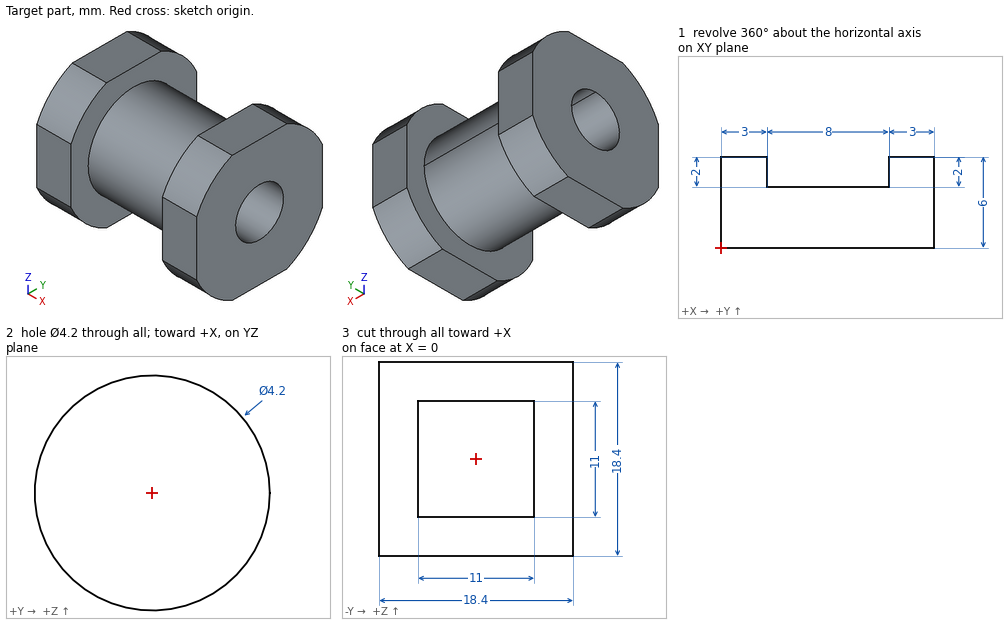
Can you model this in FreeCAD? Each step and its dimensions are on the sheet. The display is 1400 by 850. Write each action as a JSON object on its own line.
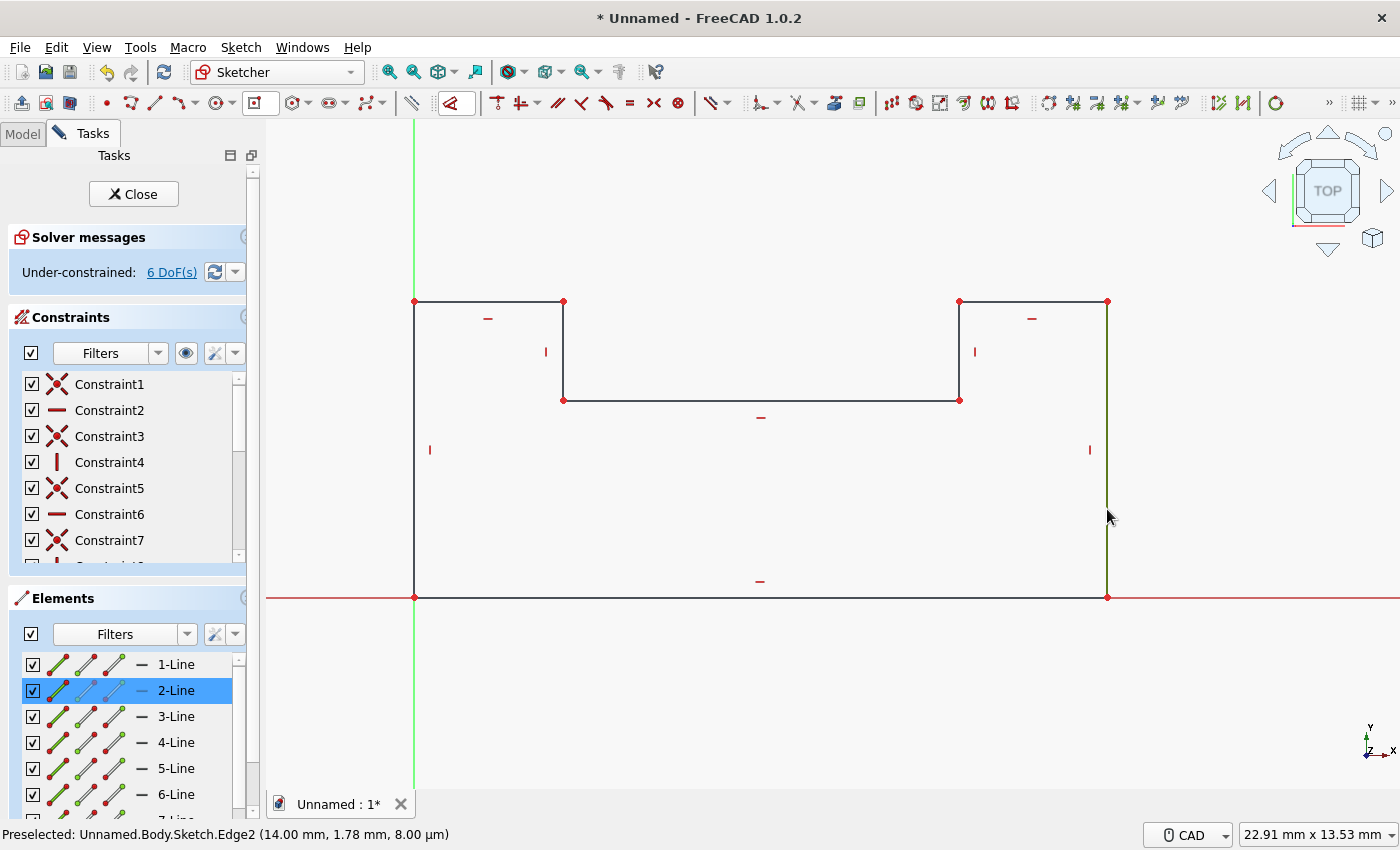
{"action": "left_click", "coordinate": [470, 104]}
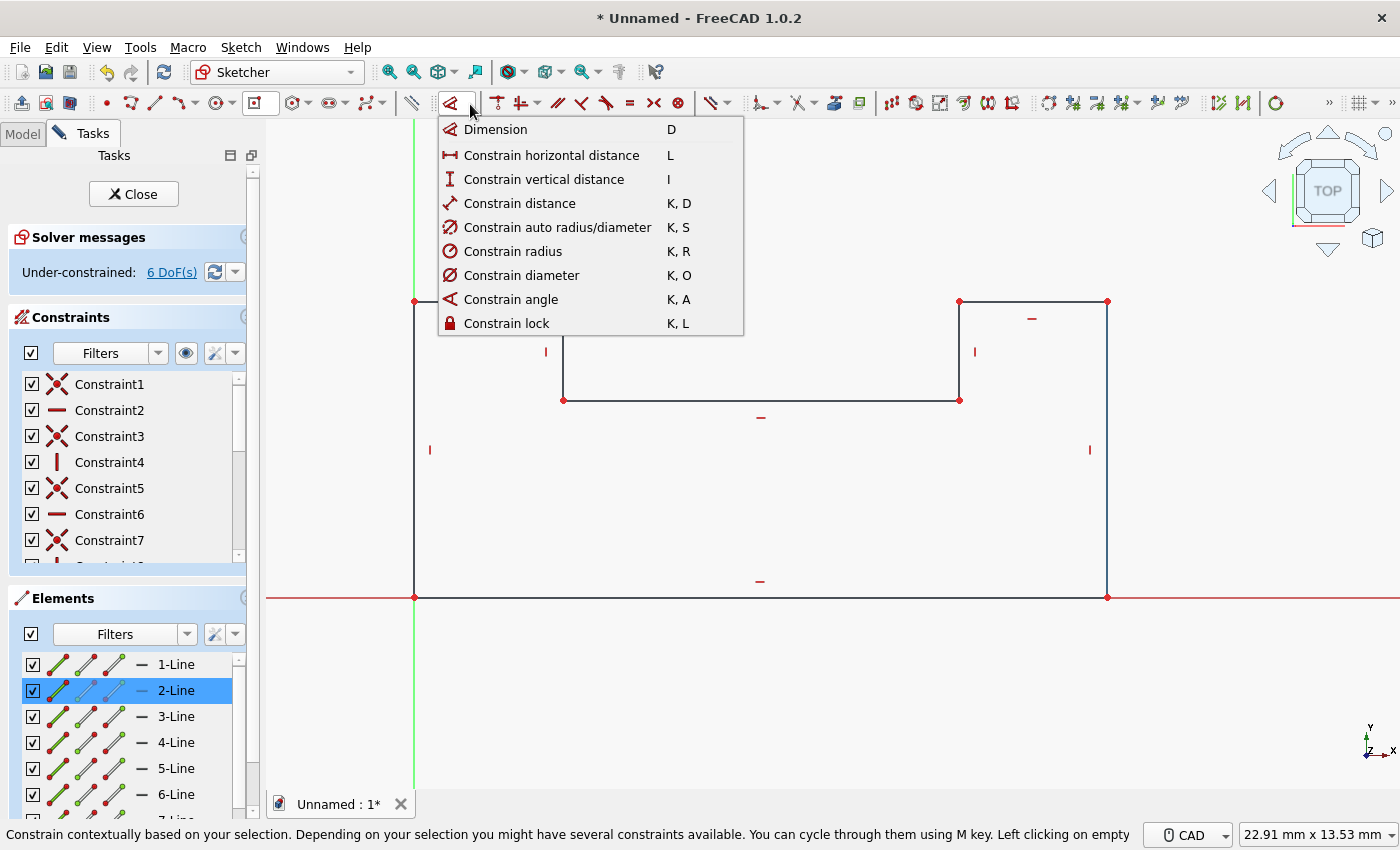
{"action": "left_click", "coordinate": [591, 179]}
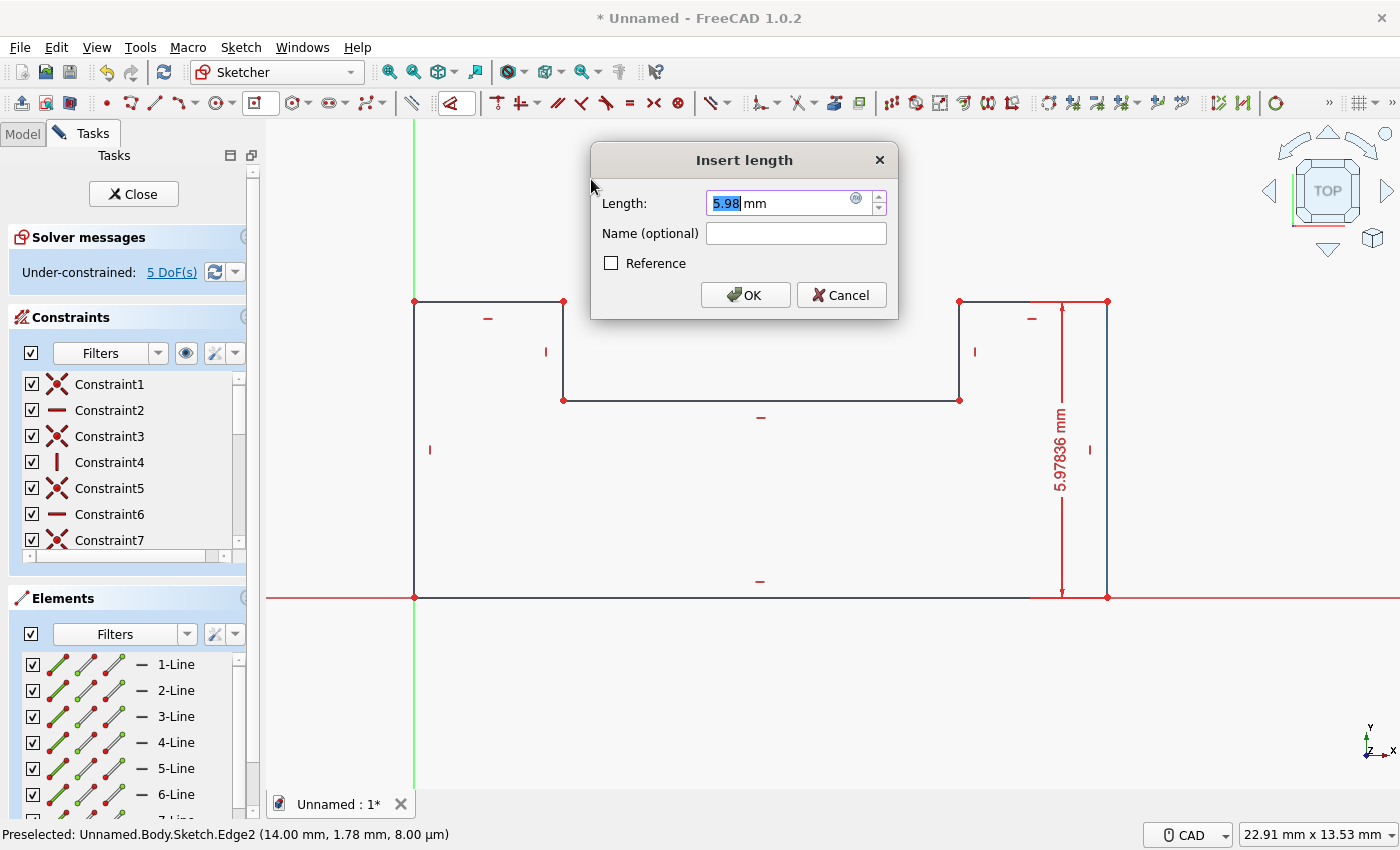
{"action": "type", "text": "6"}
{"action": "key", "text": "Return"}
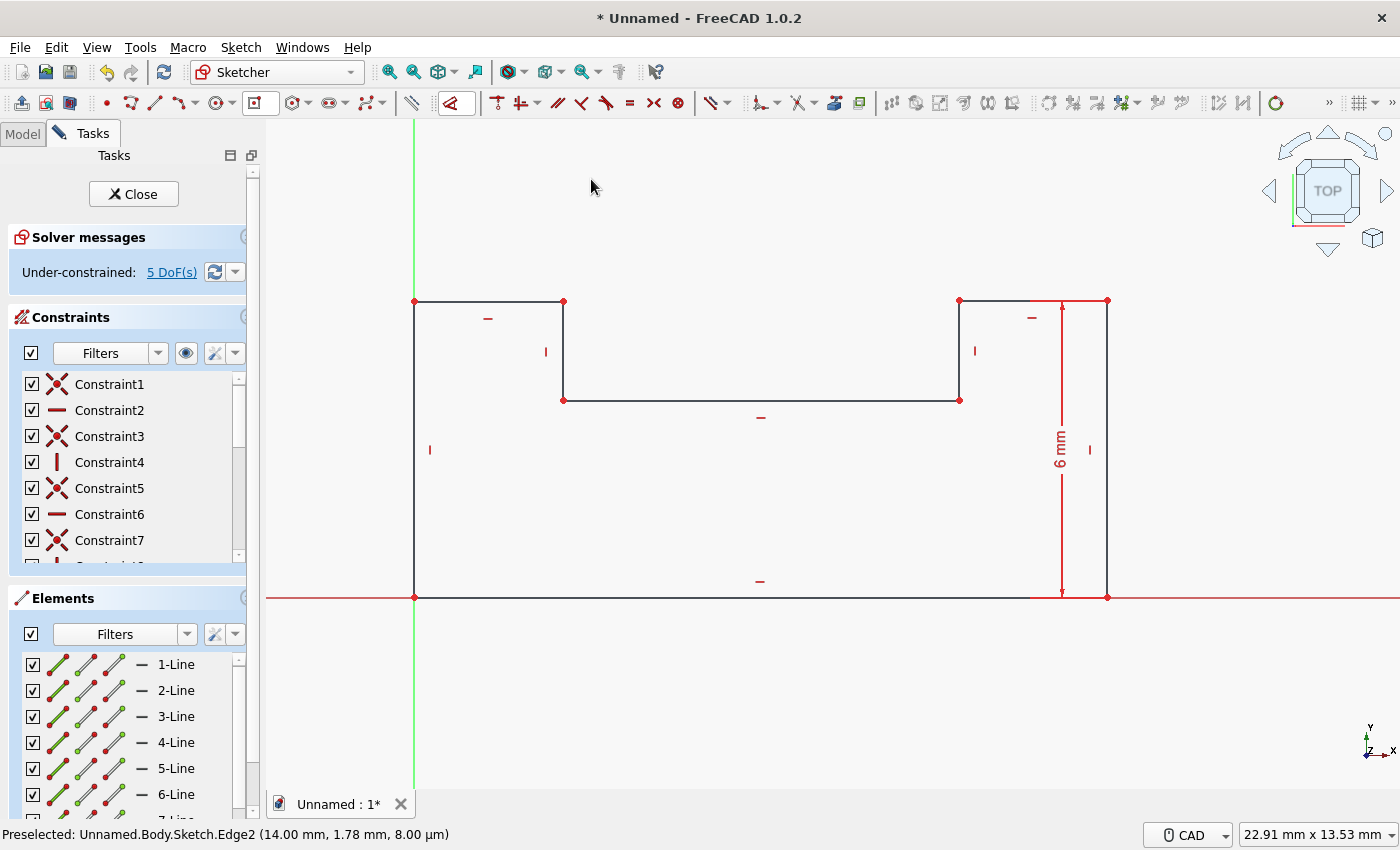
{"action": "left_click", "coordinate": [1063, 301]}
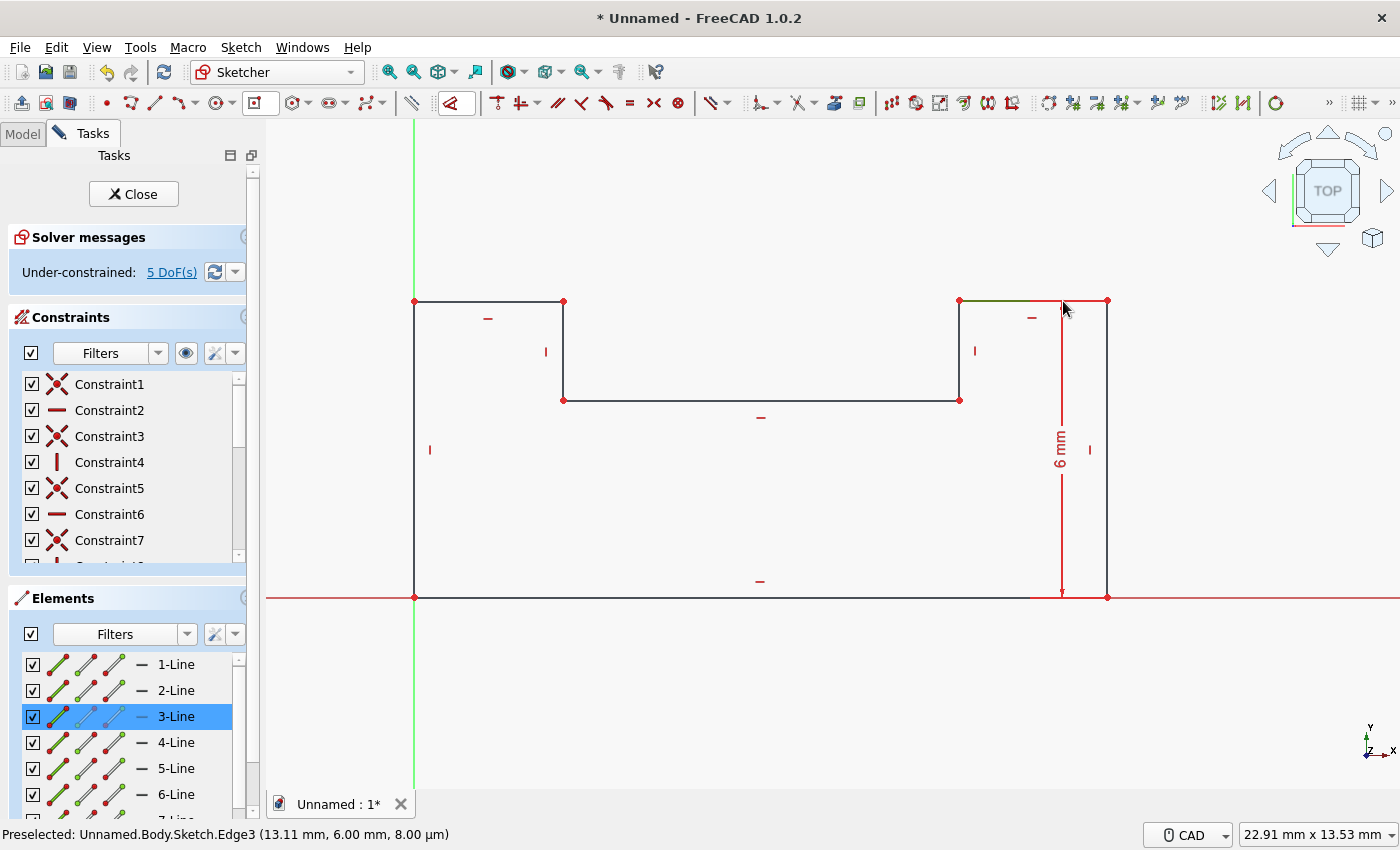
{"action": "left_click", "coordinate": [470, 104]}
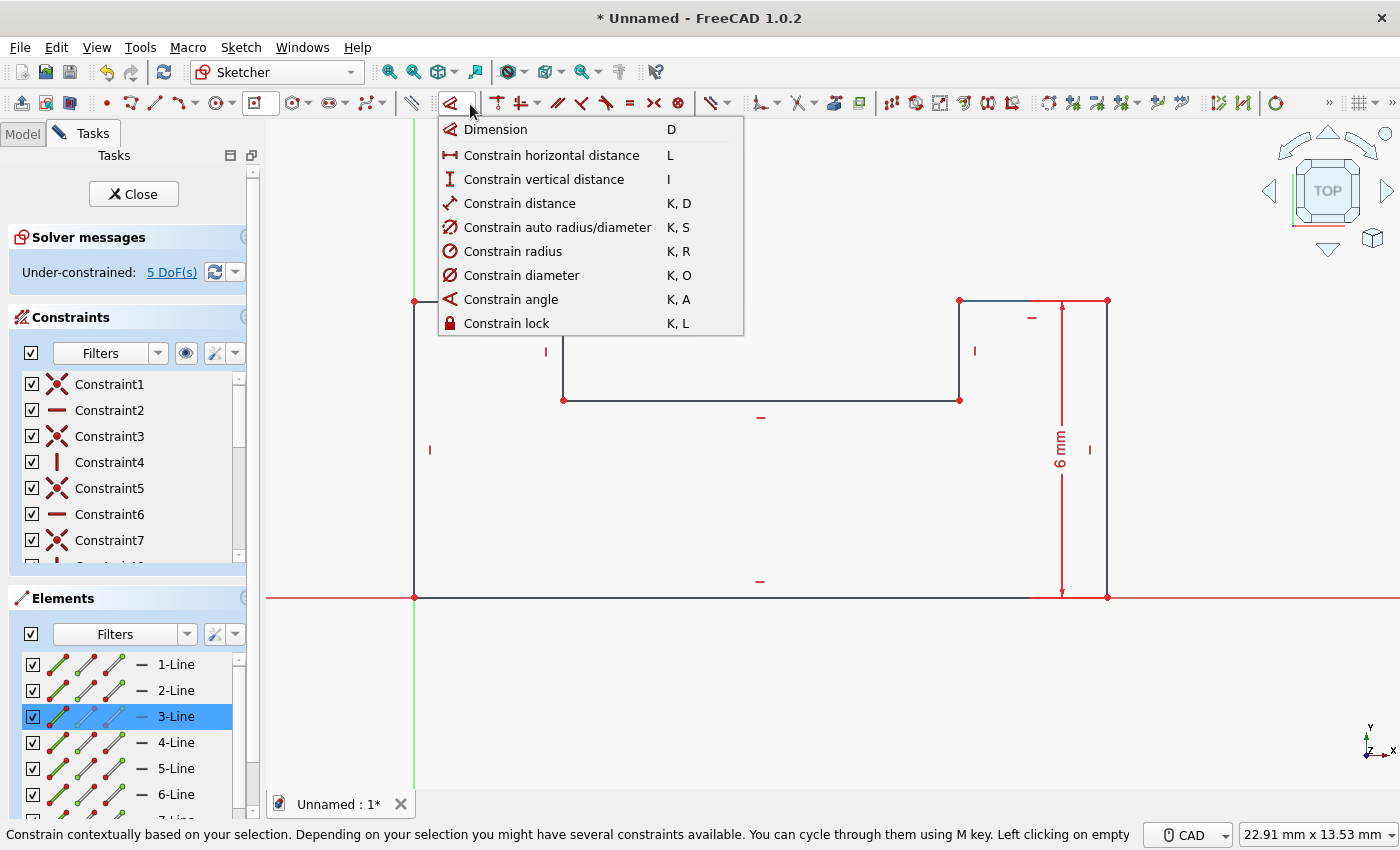
{"action": "left_click", "coordinate": [591, 155]}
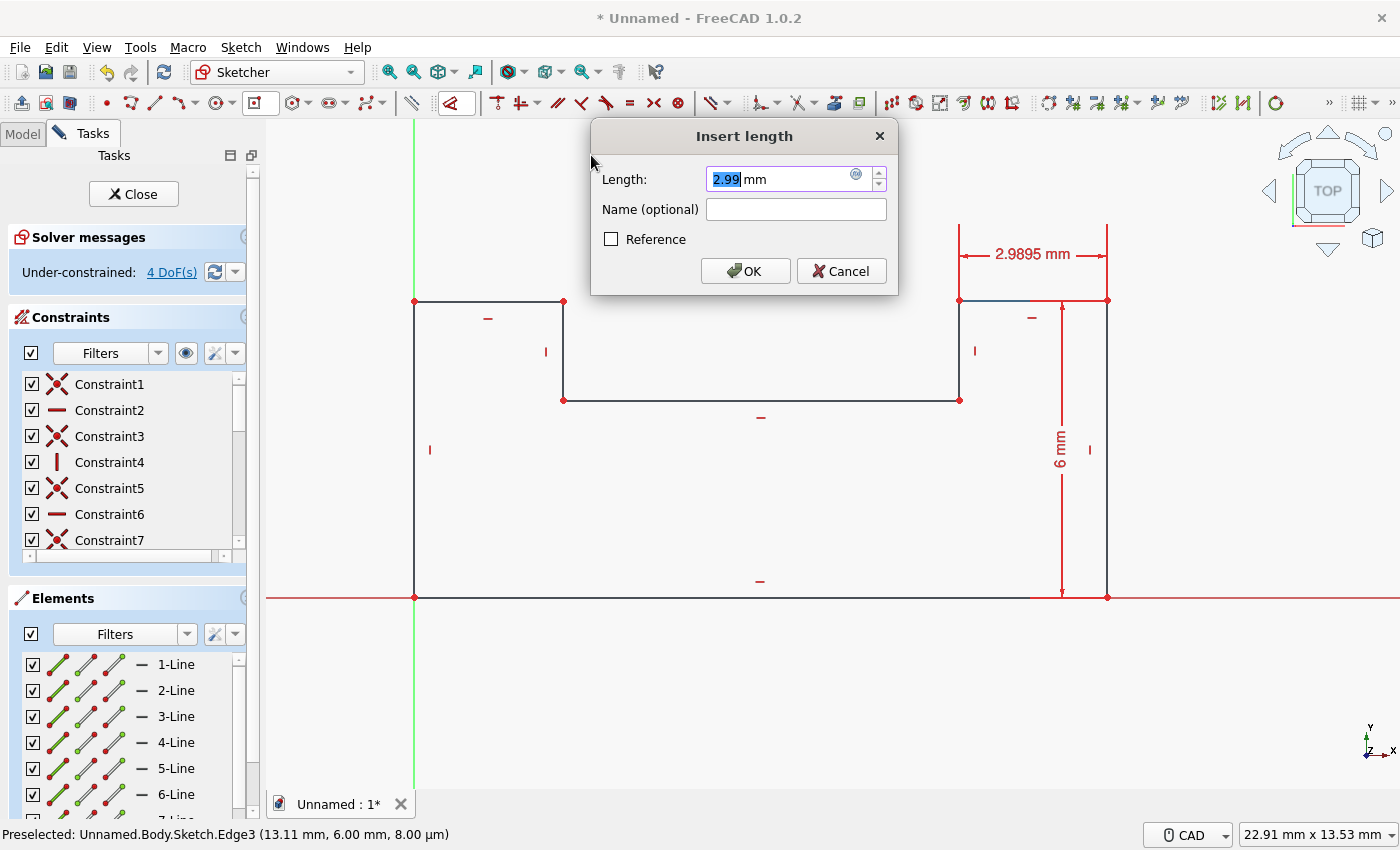
{"action": "type", "text": "3"}
{"action": "key", "text": "Return"}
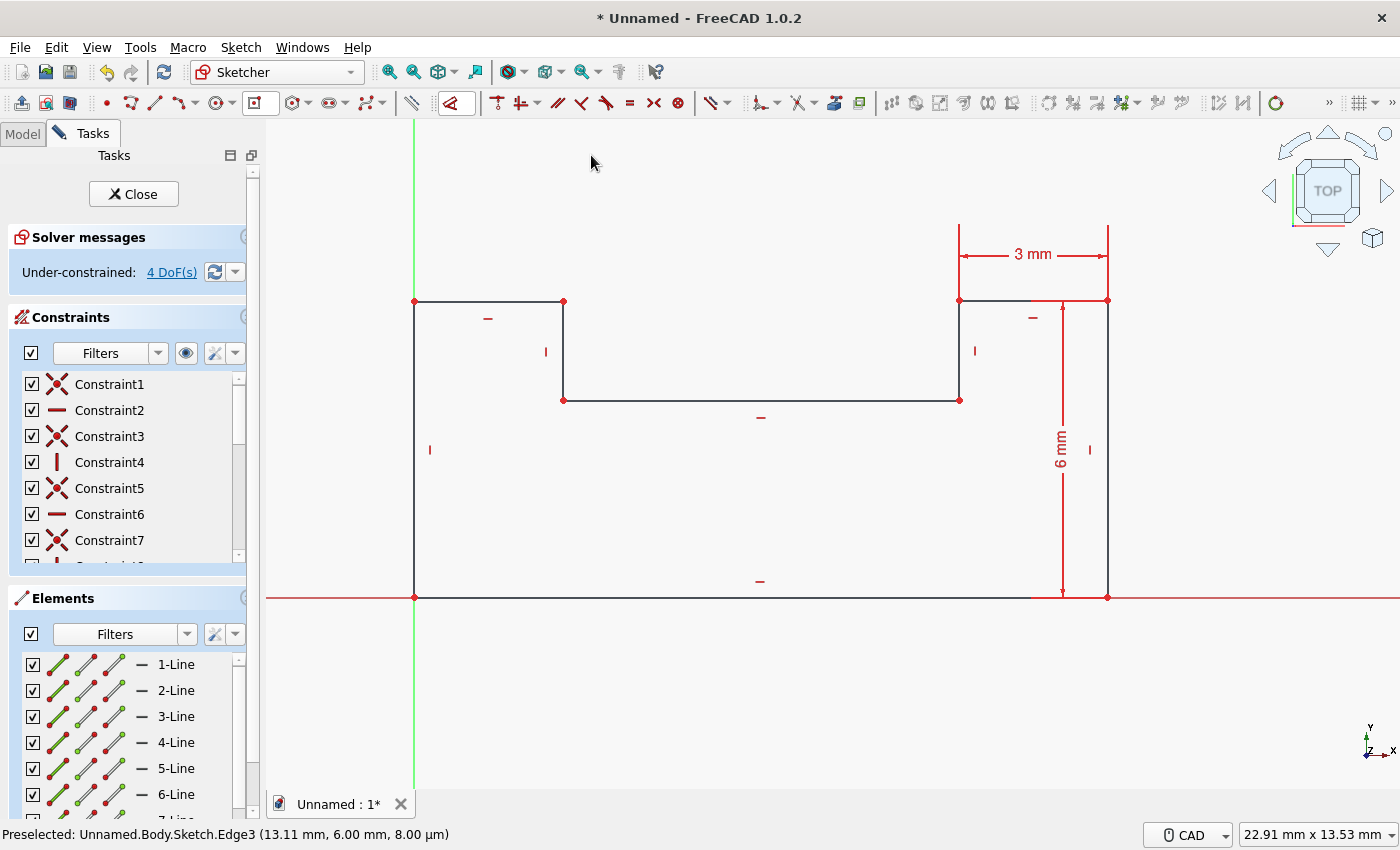
{"action": "left_click", "coordinate": [959, 331]}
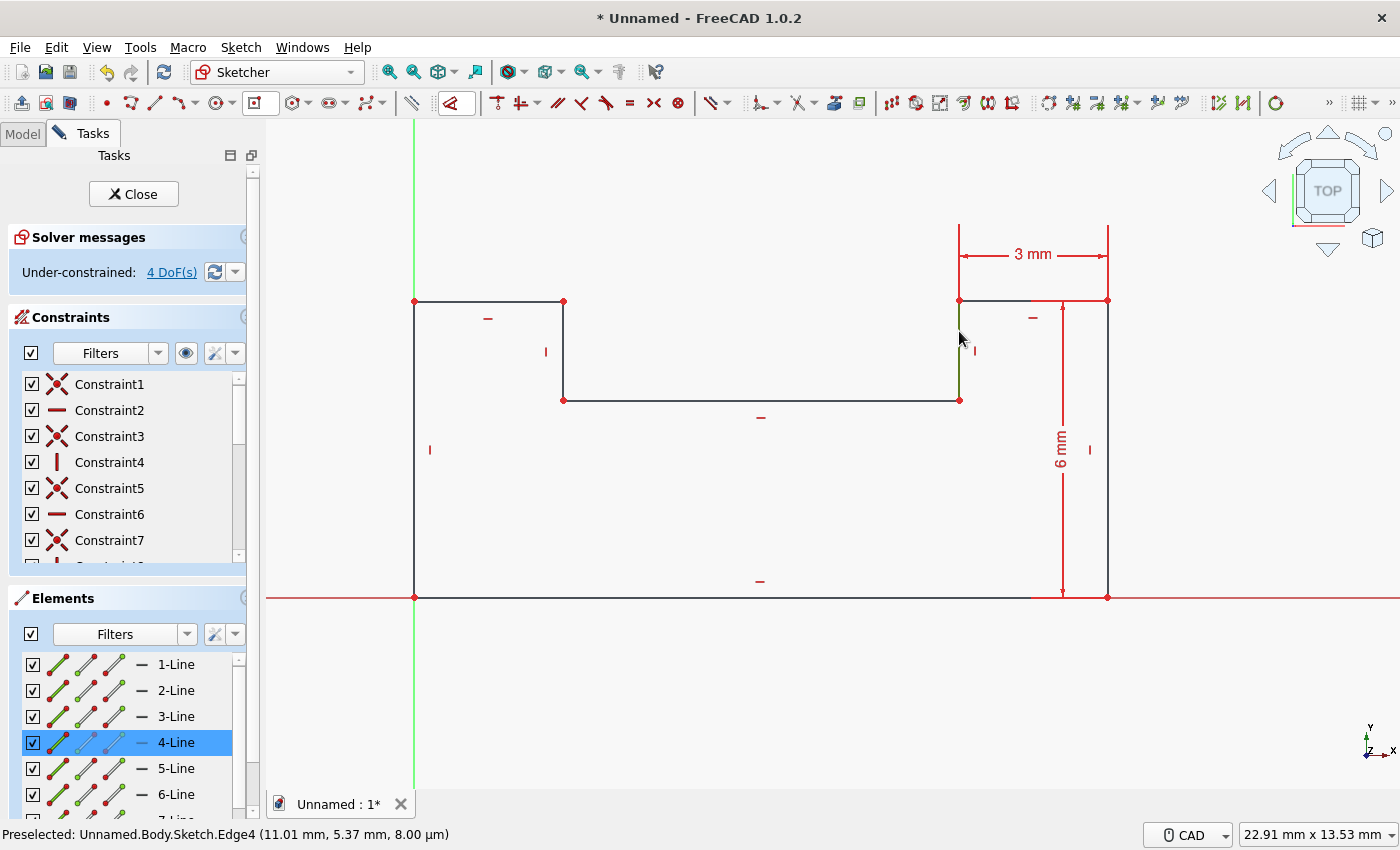
{"action": "left_click", "coordinate": [470, 104]}